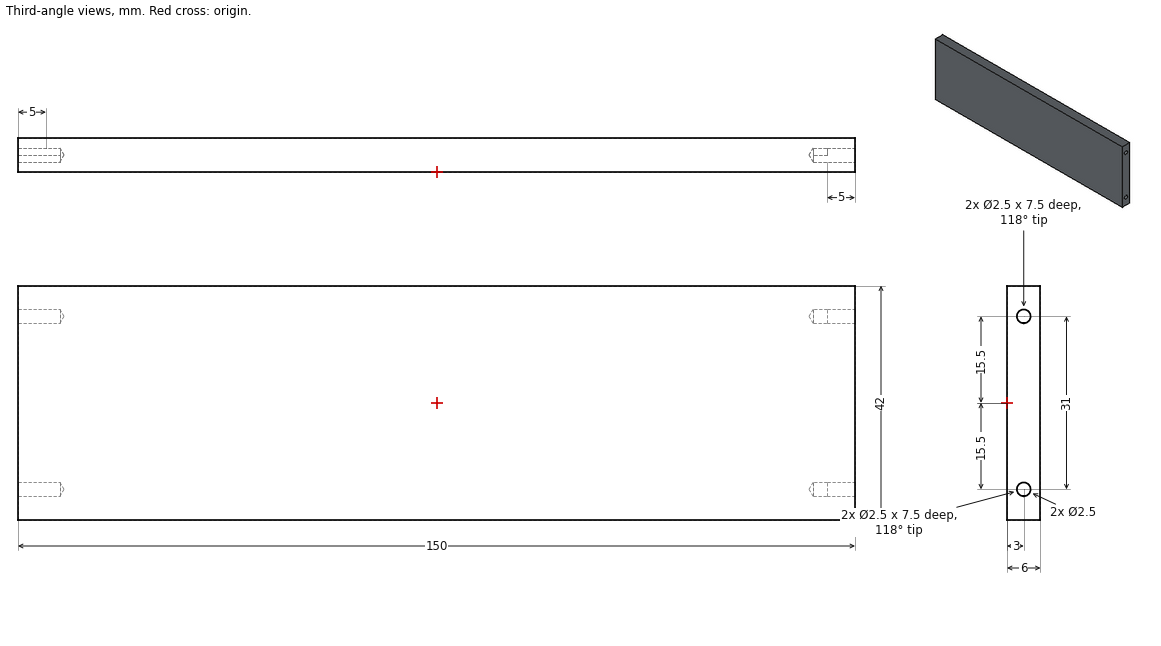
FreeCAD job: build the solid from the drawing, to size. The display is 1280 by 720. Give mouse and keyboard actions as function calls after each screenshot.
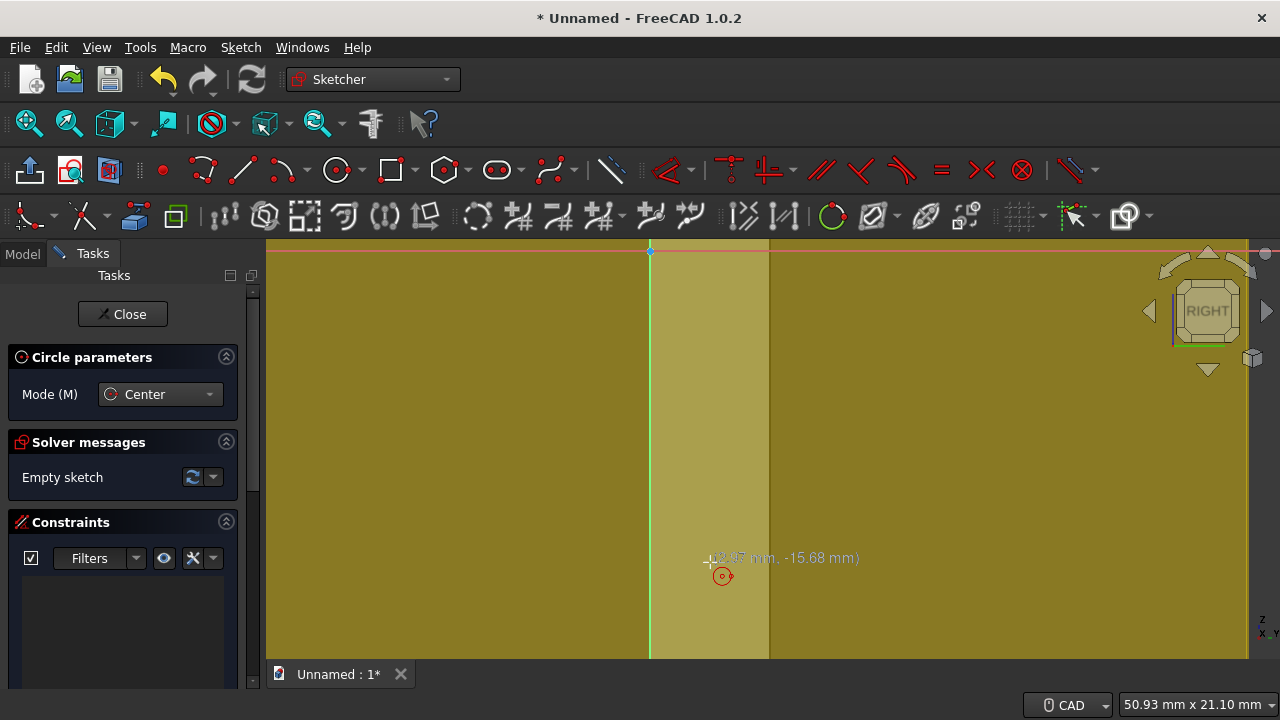
click(710, 560)
move(727, 542)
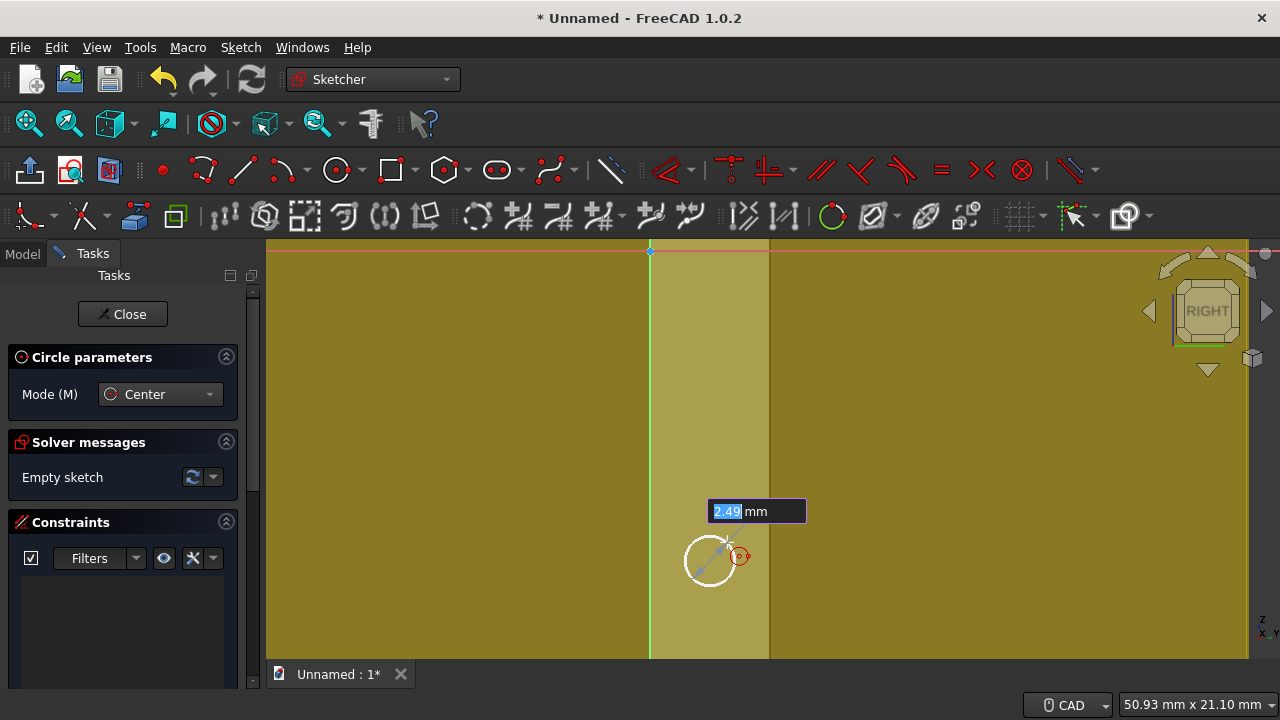
text(2.5)
key(Return)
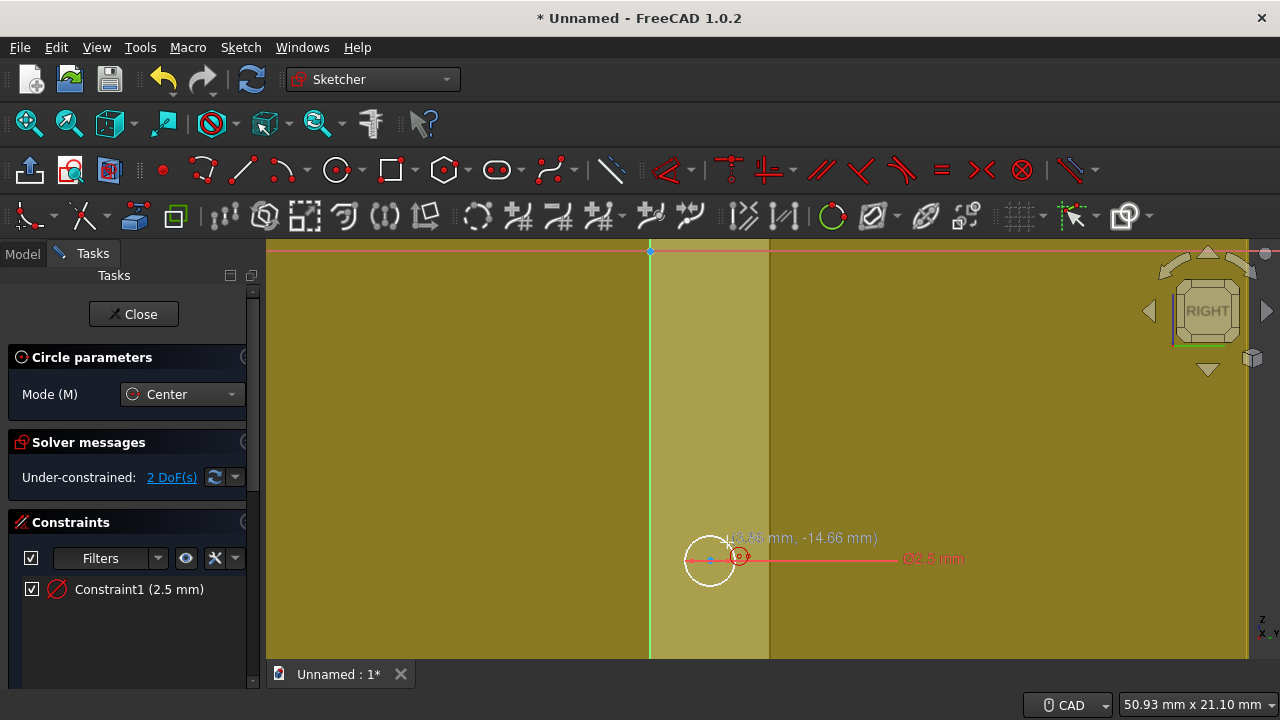
scroll(712, 564, down, 5)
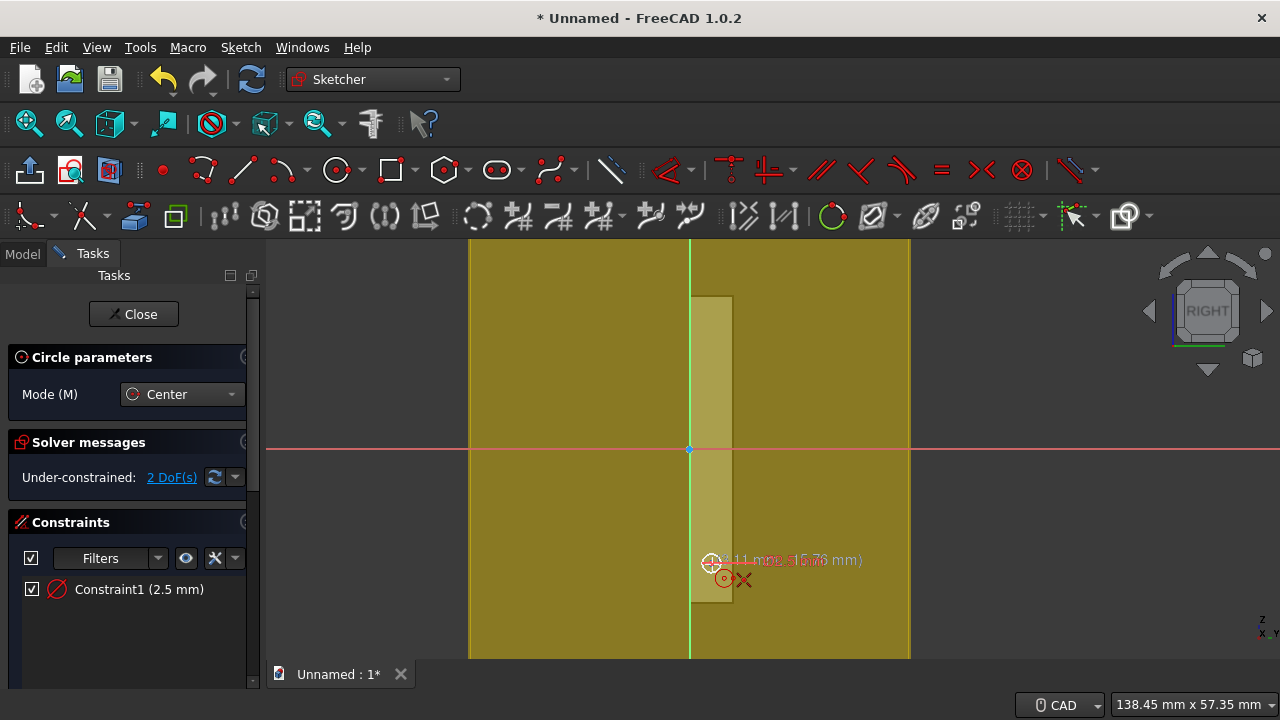
scroll(711, 336, up, 5)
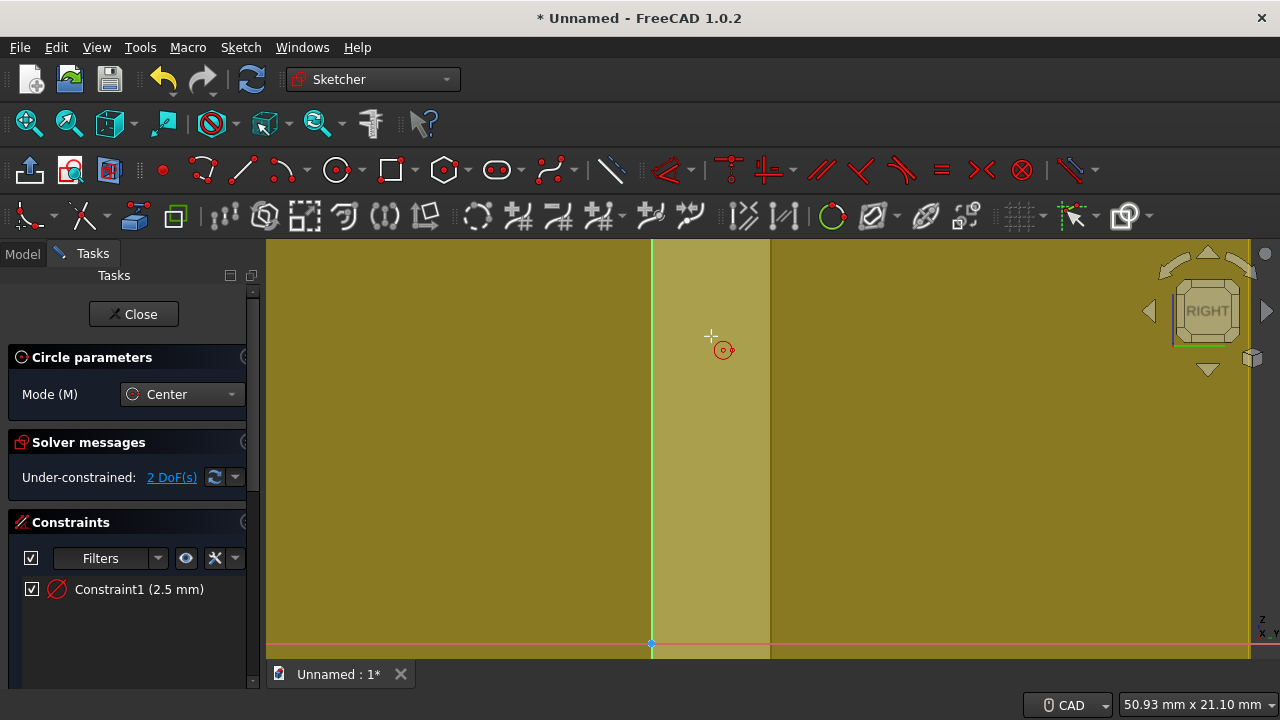
click(712, 335)
move(729, 318)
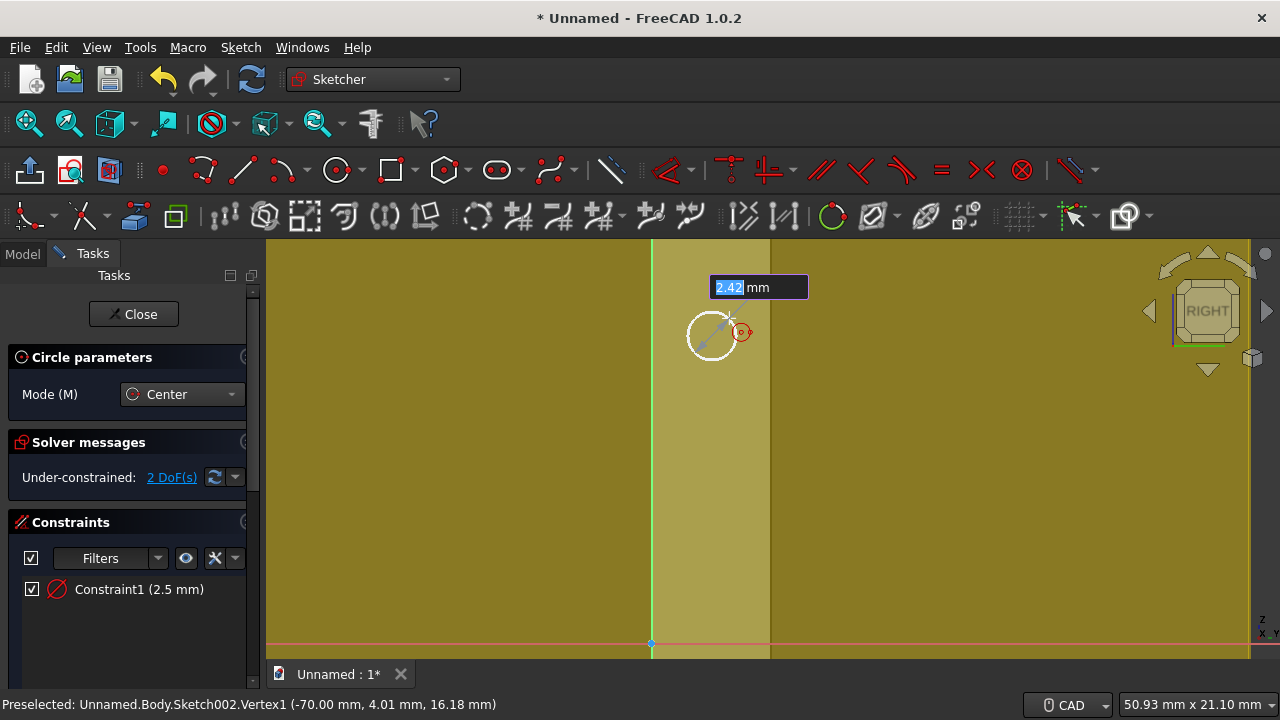
text(2.5)
key(Return)
key(Escape)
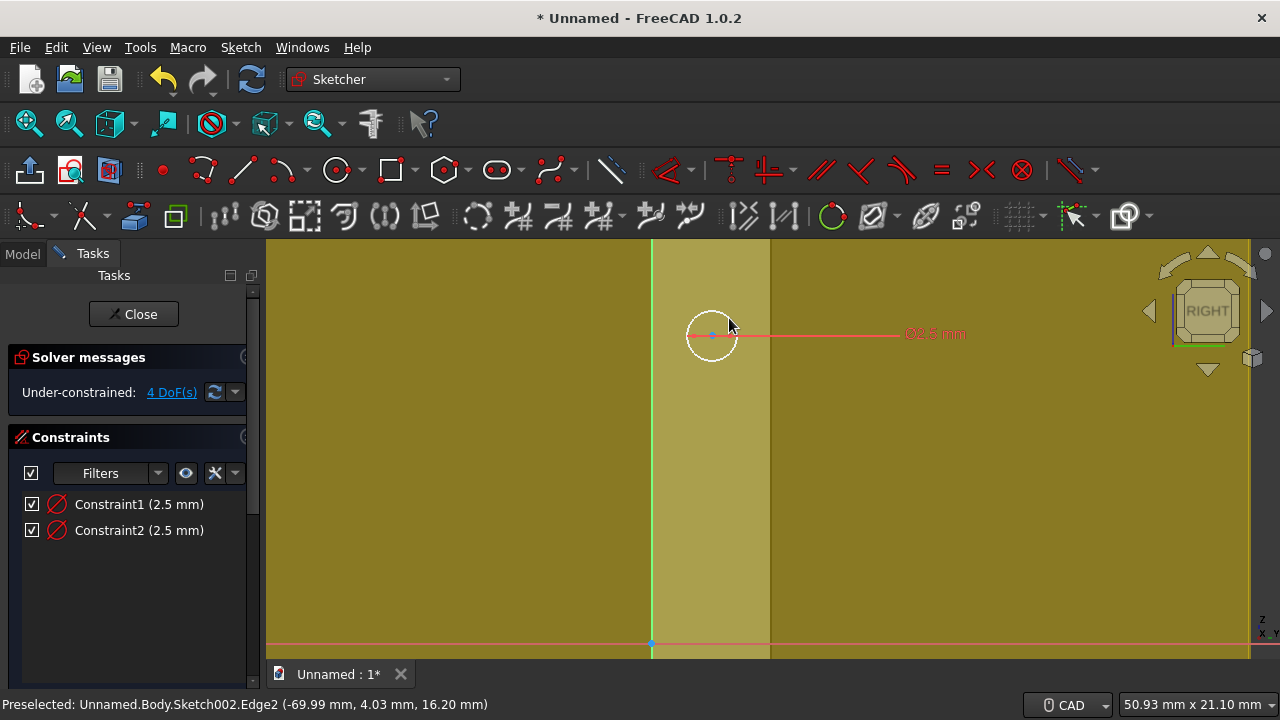
scroll(711, 336, down, 5)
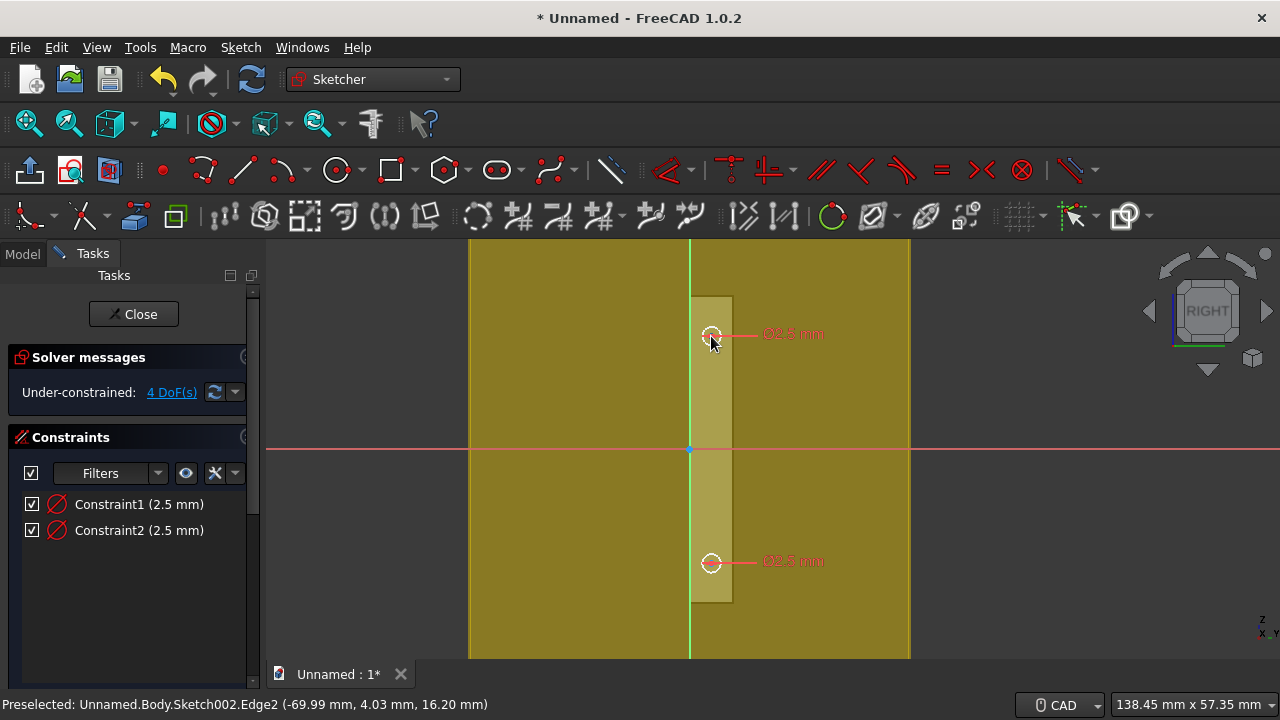
click(712, 563)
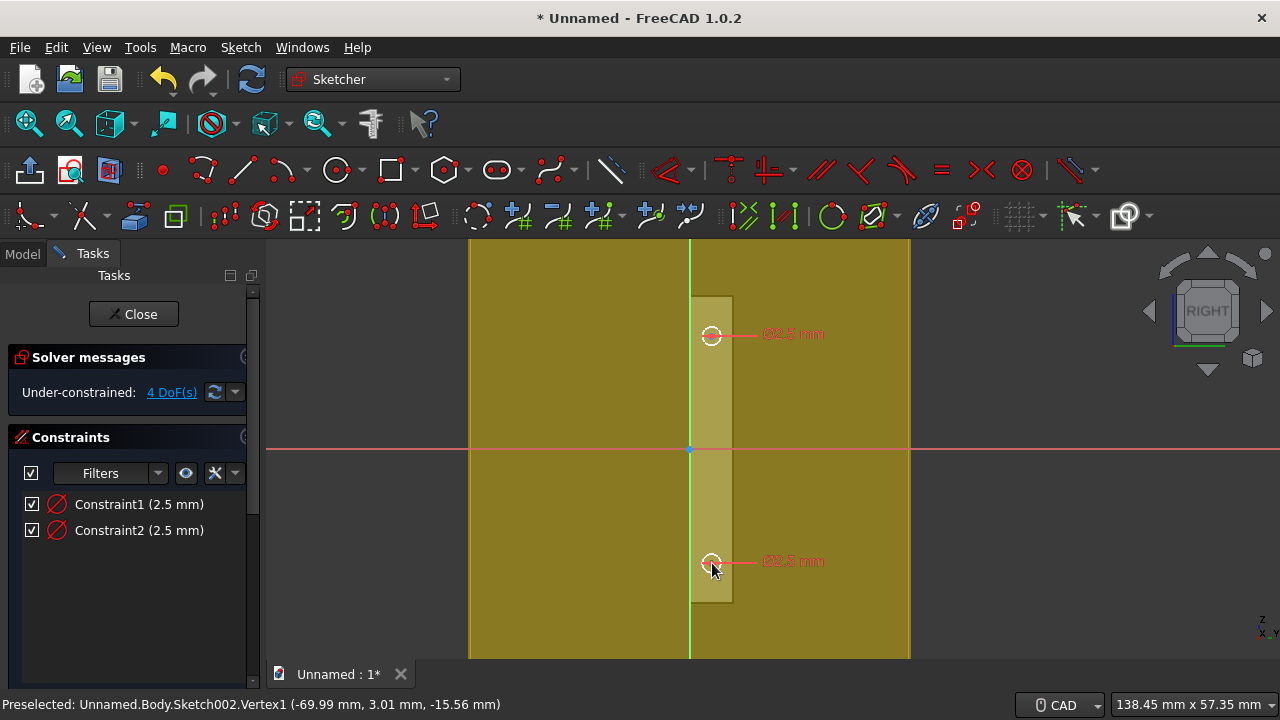
click(712, 336)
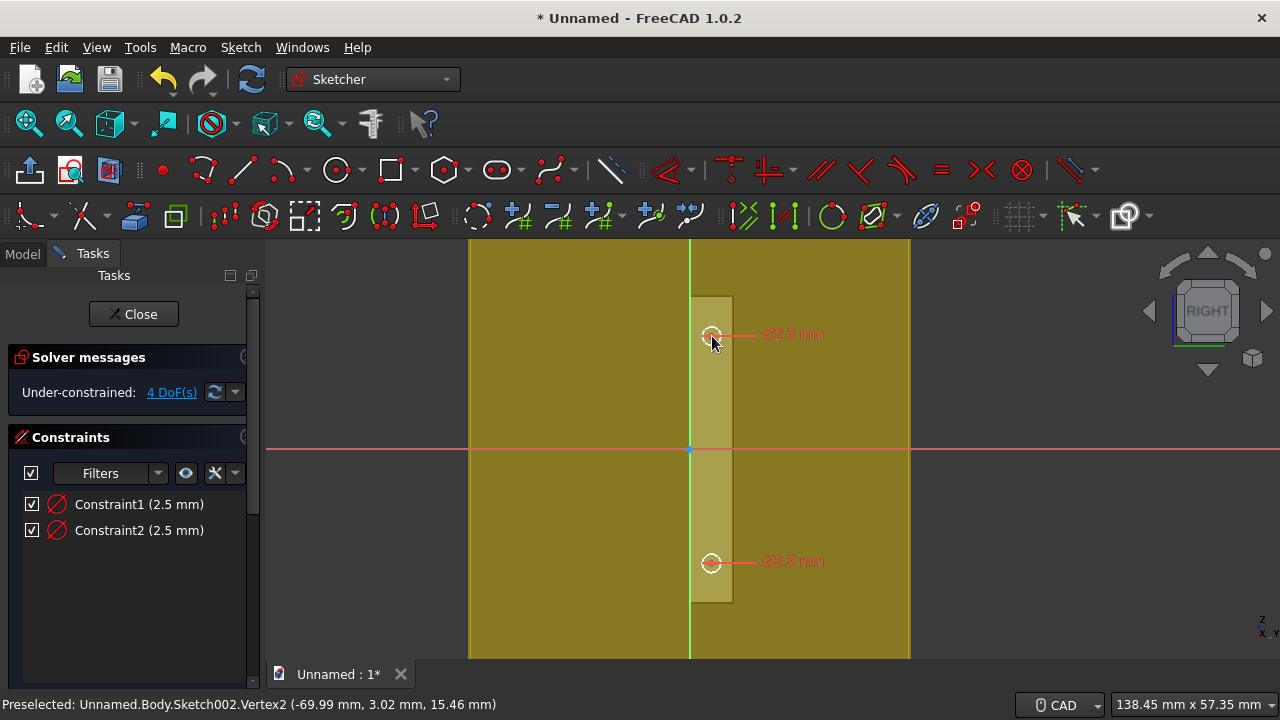
click(796, 170)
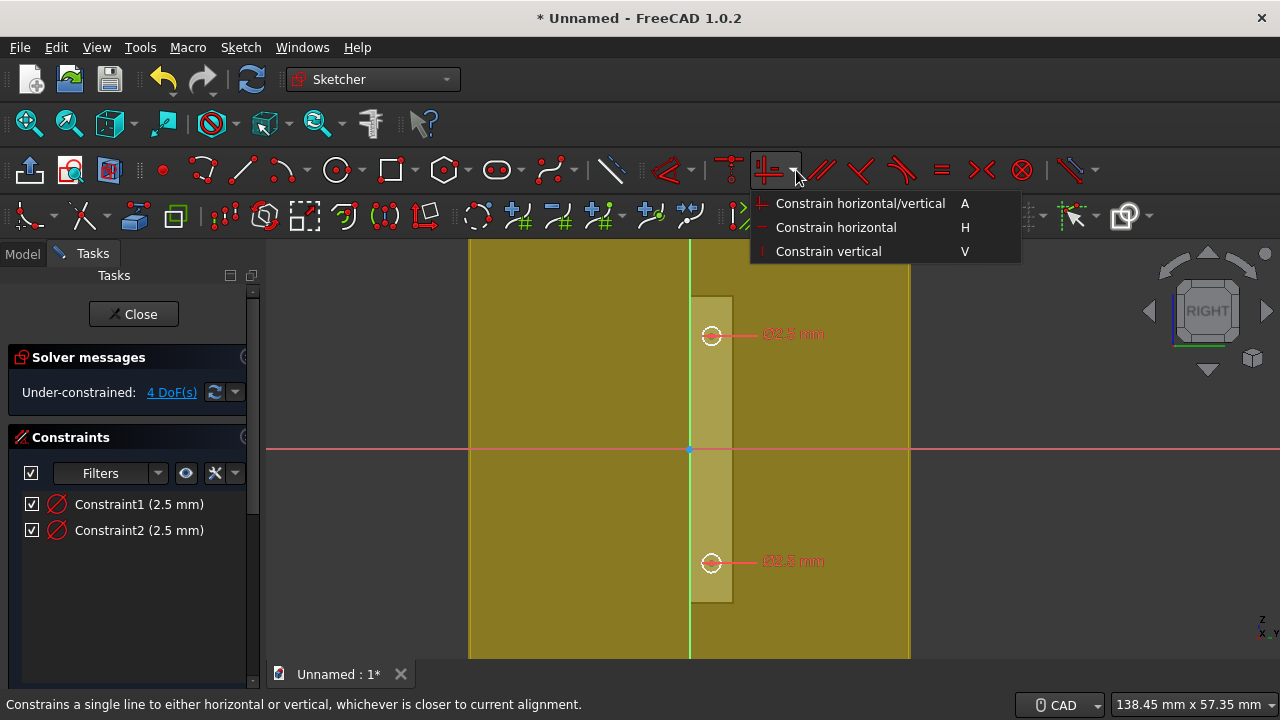
click(886, 251)